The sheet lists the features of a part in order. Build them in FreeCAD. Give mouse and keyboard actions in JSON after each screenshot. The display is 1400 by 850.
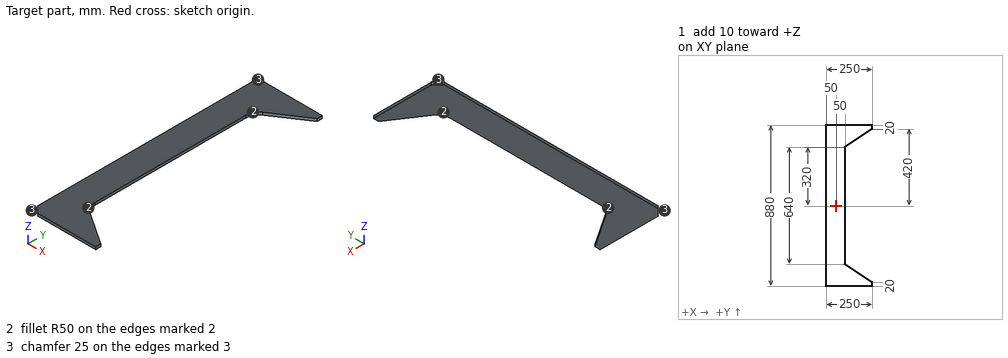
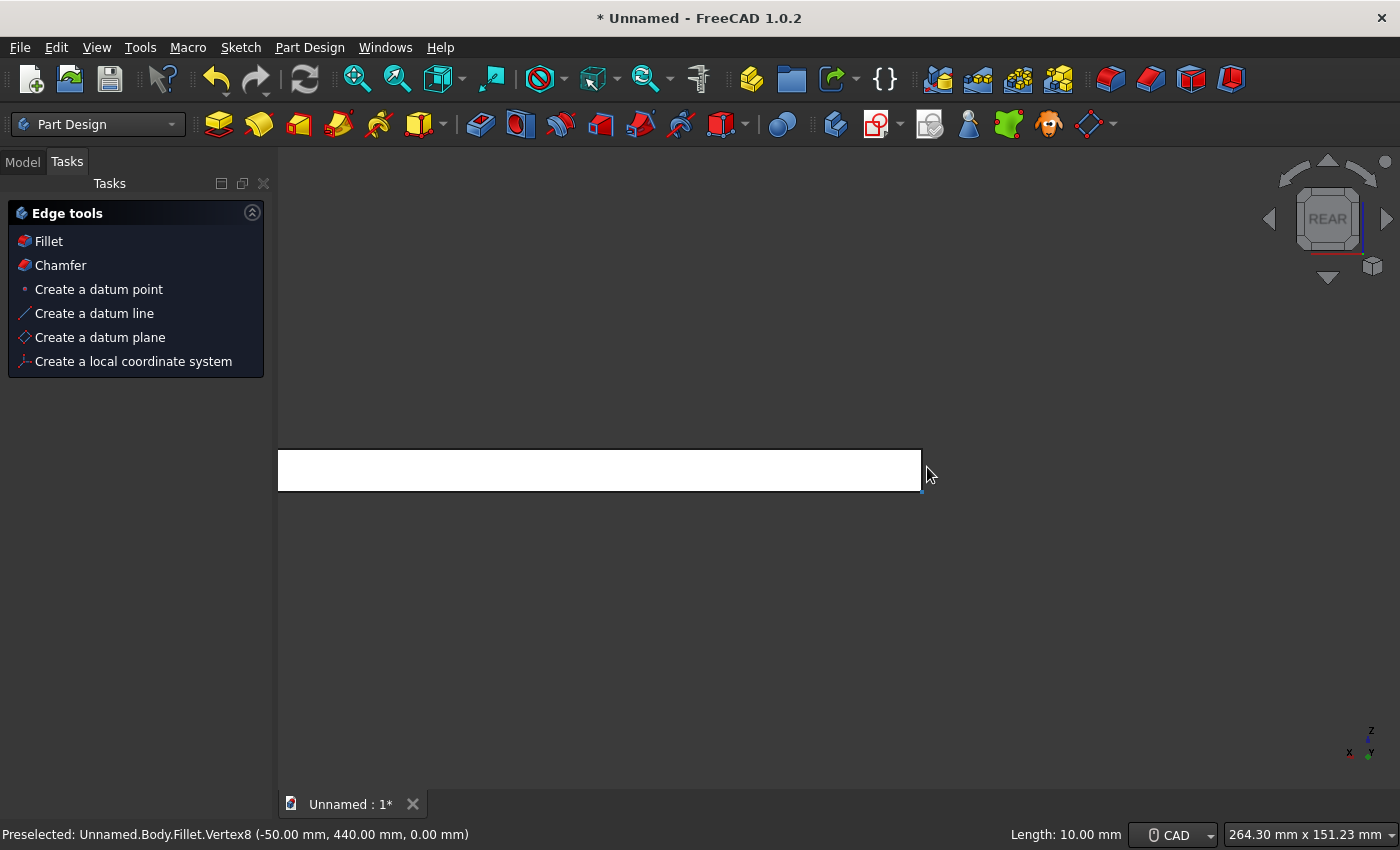
{"action": "left_click", "coordinate": [922, 470], "text": "ctrl"}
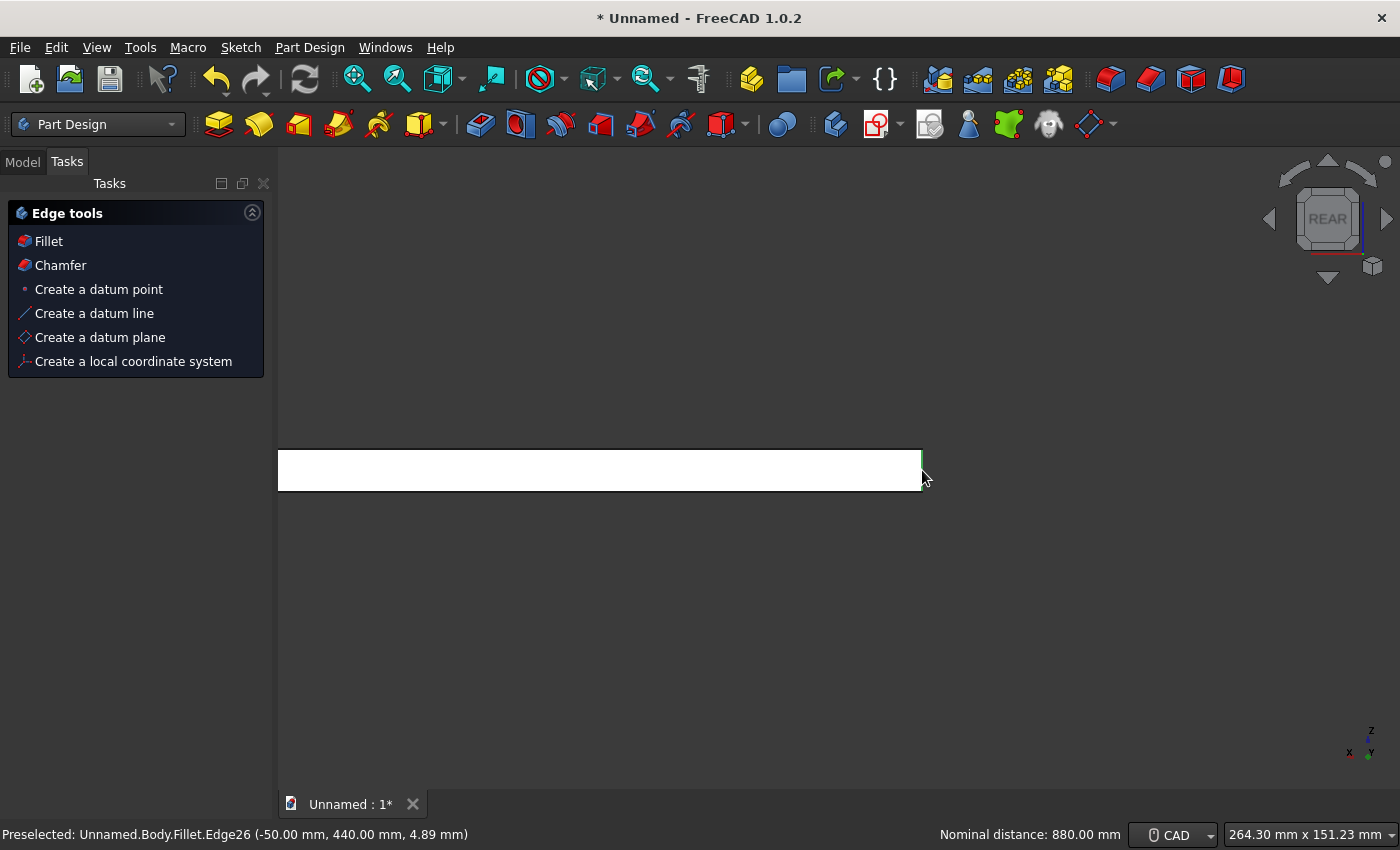
{"action": "left_click", "coordinate": [1152, 80]}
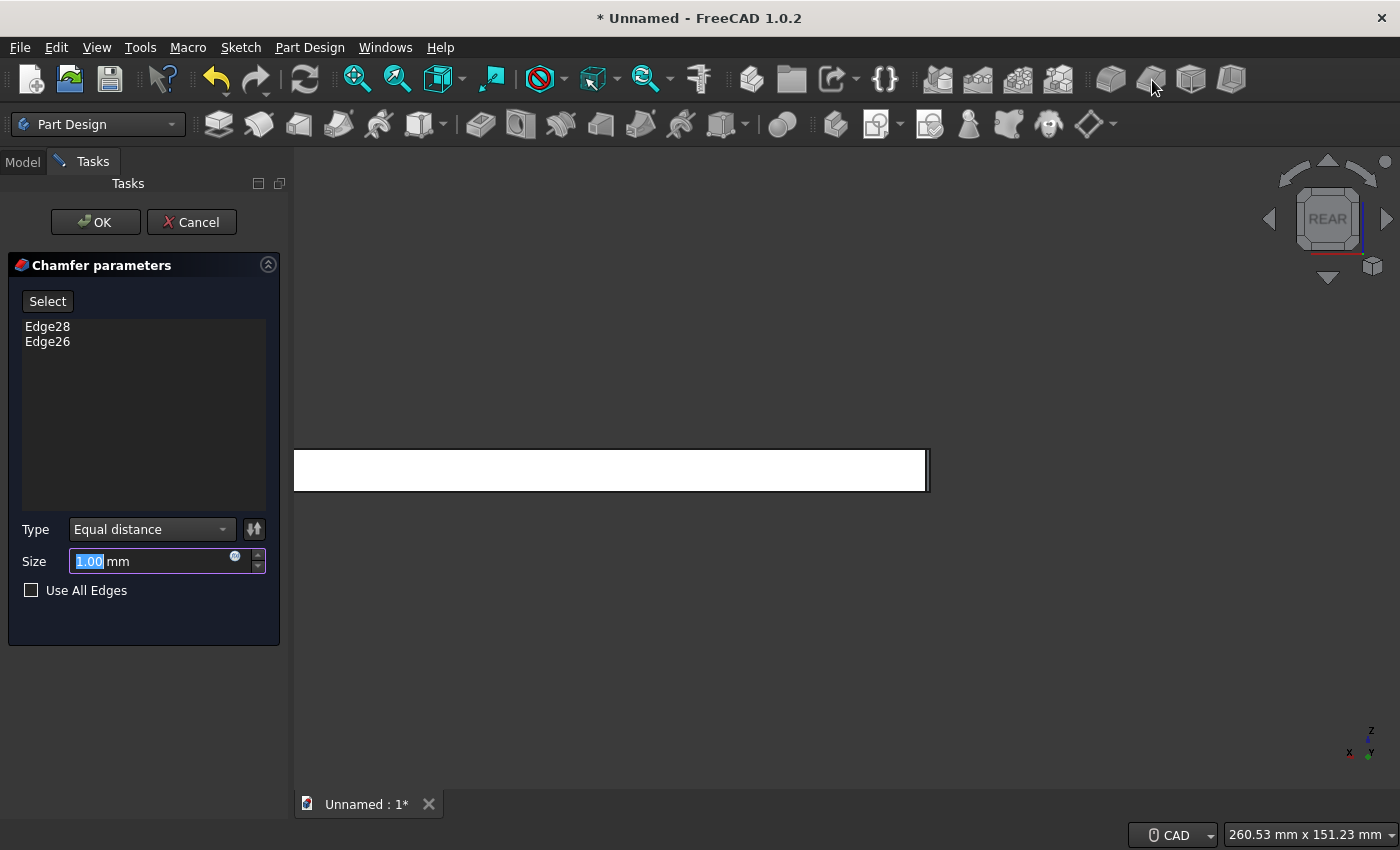
{"action": "type", "text": "25"}
{"action": "key", "text": "Tab"}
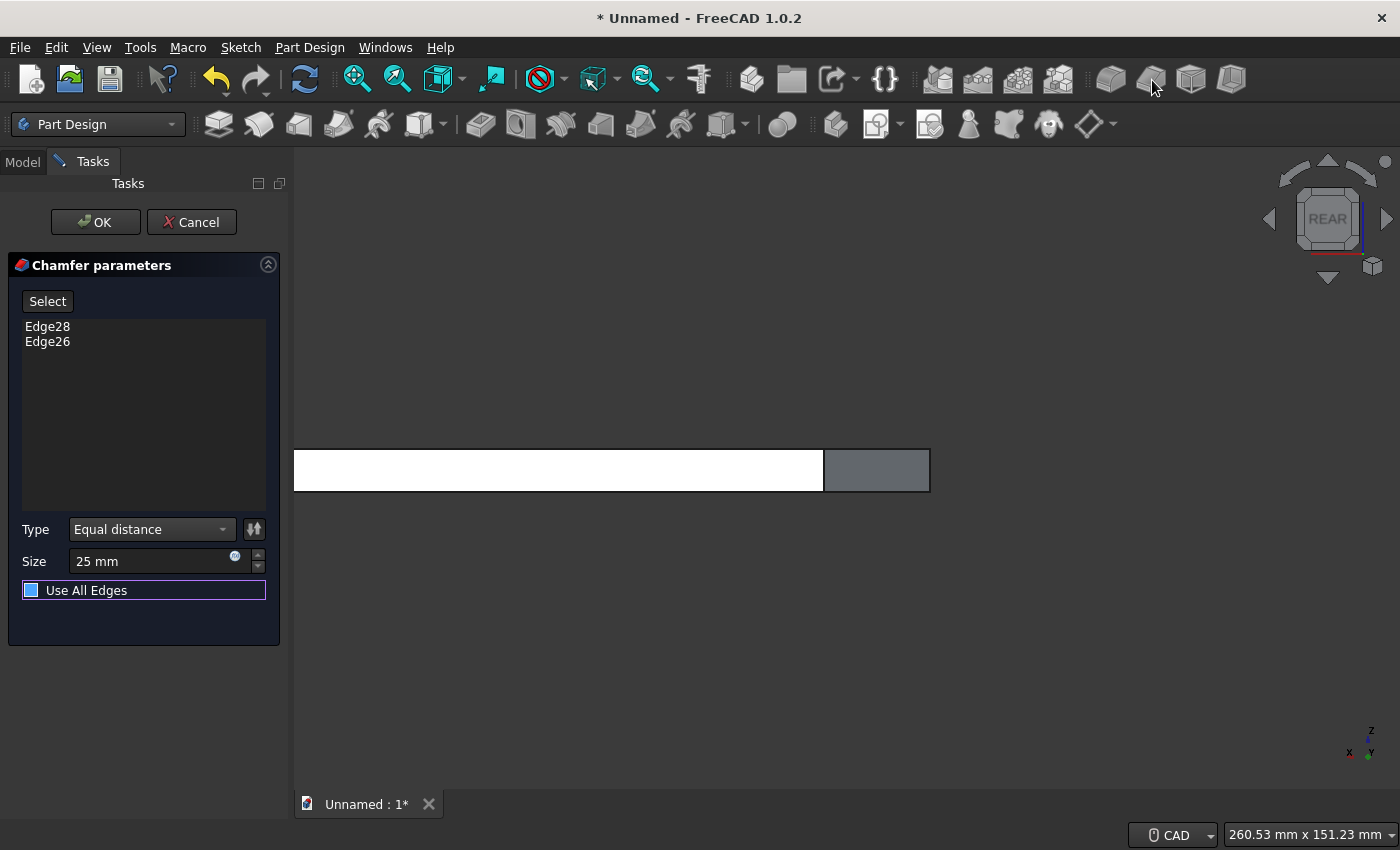
{"action": "left_click", "coordinate": [96, 222]}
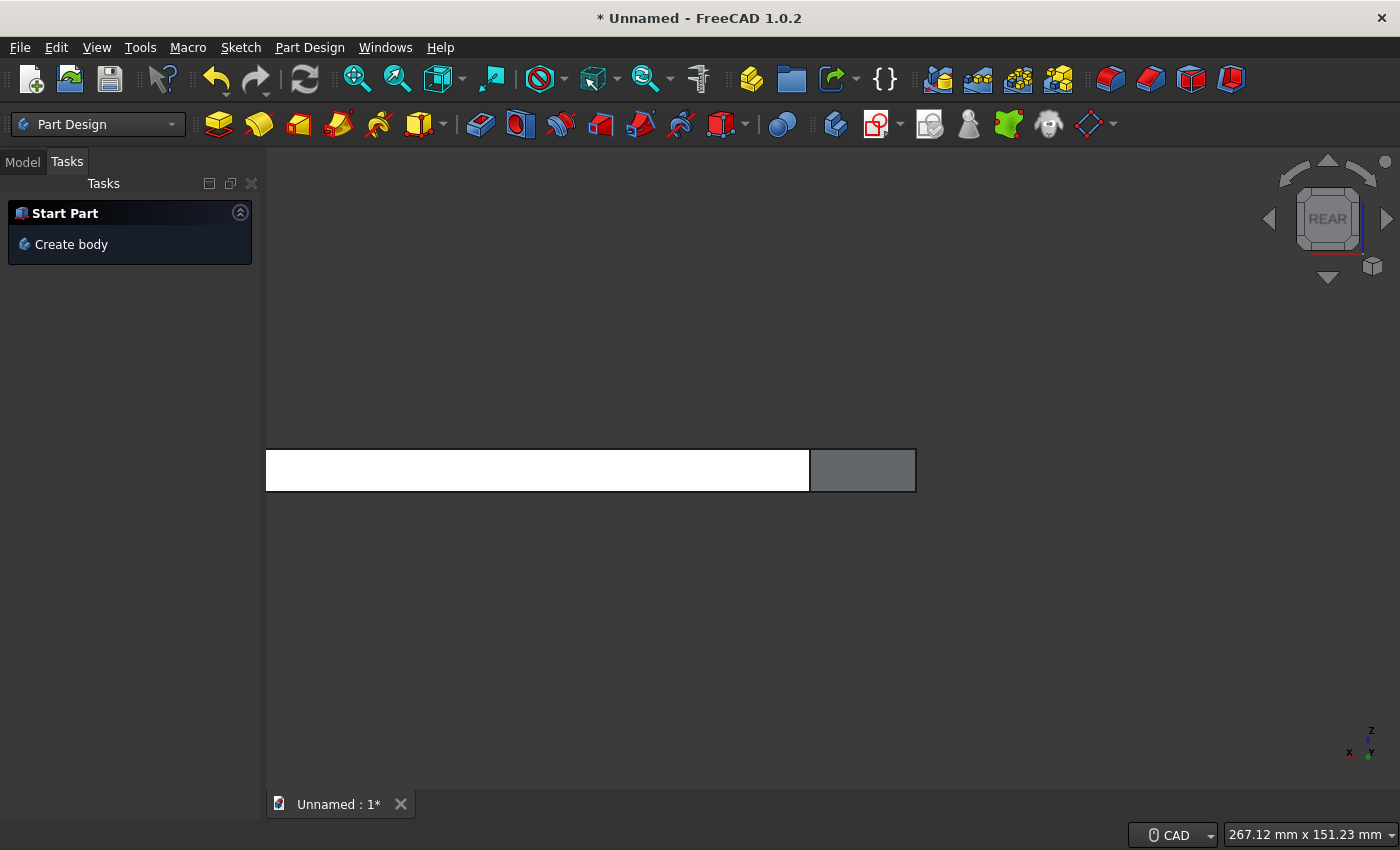
{"action": "key", "text": "0"}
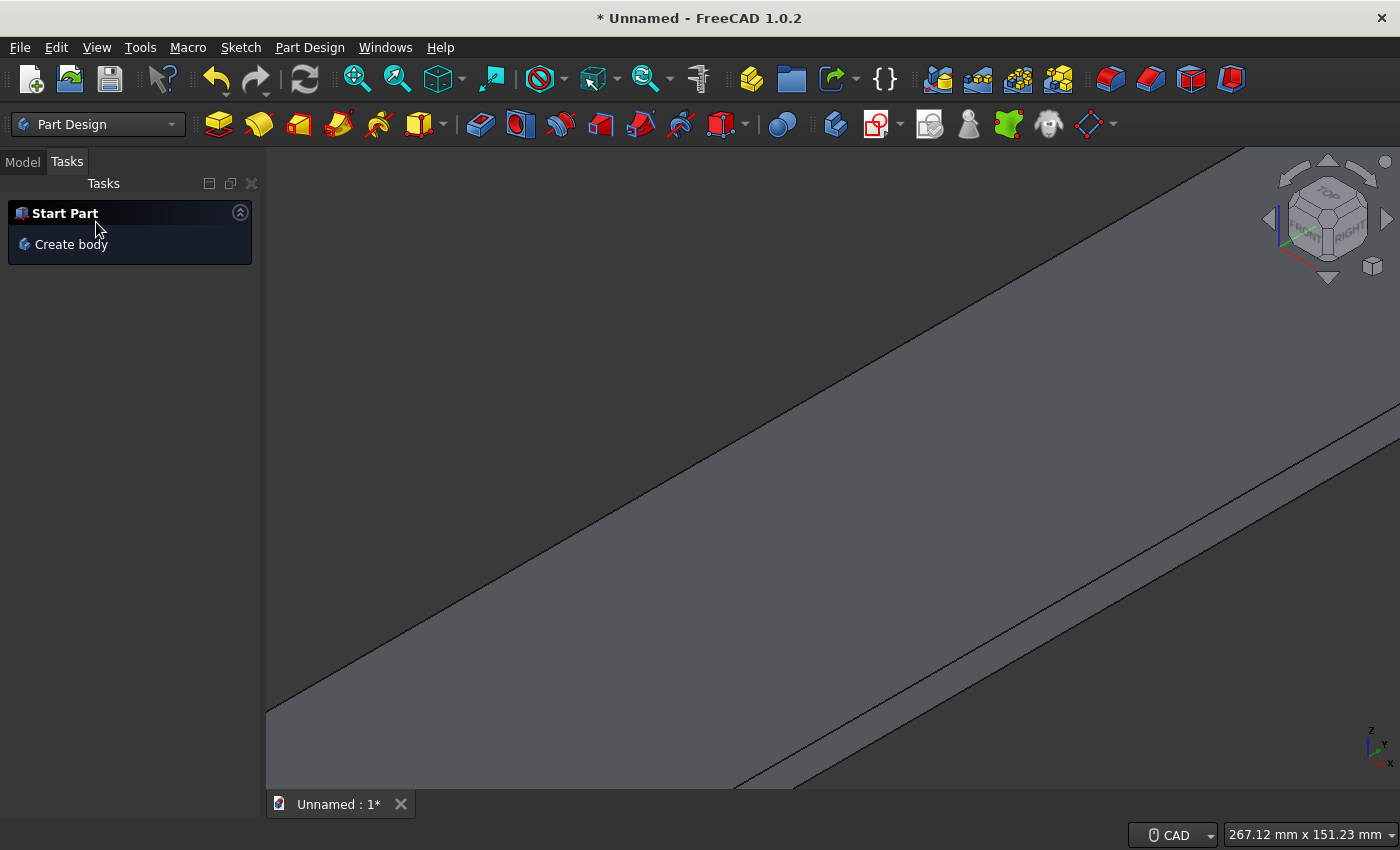
{"action": "key", "text": "v f"}